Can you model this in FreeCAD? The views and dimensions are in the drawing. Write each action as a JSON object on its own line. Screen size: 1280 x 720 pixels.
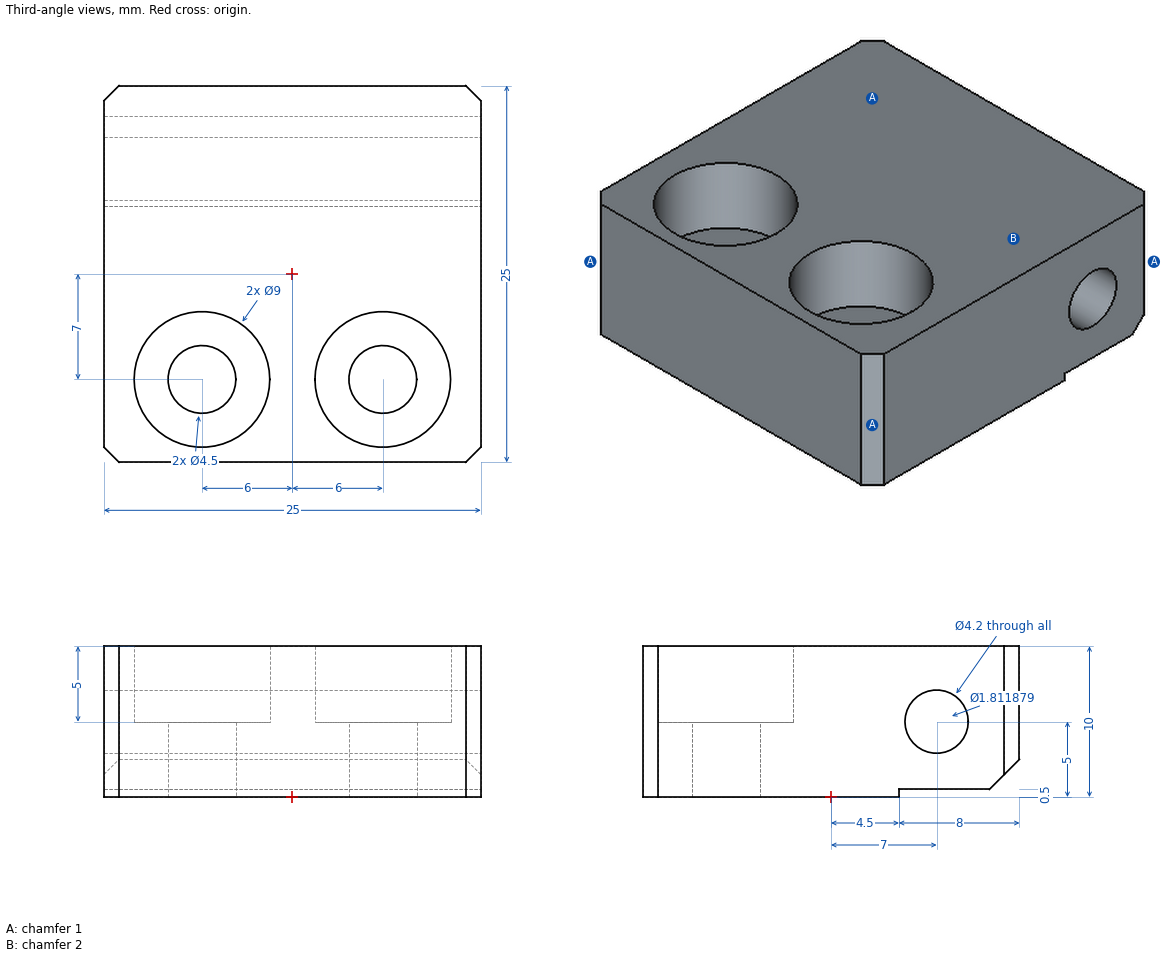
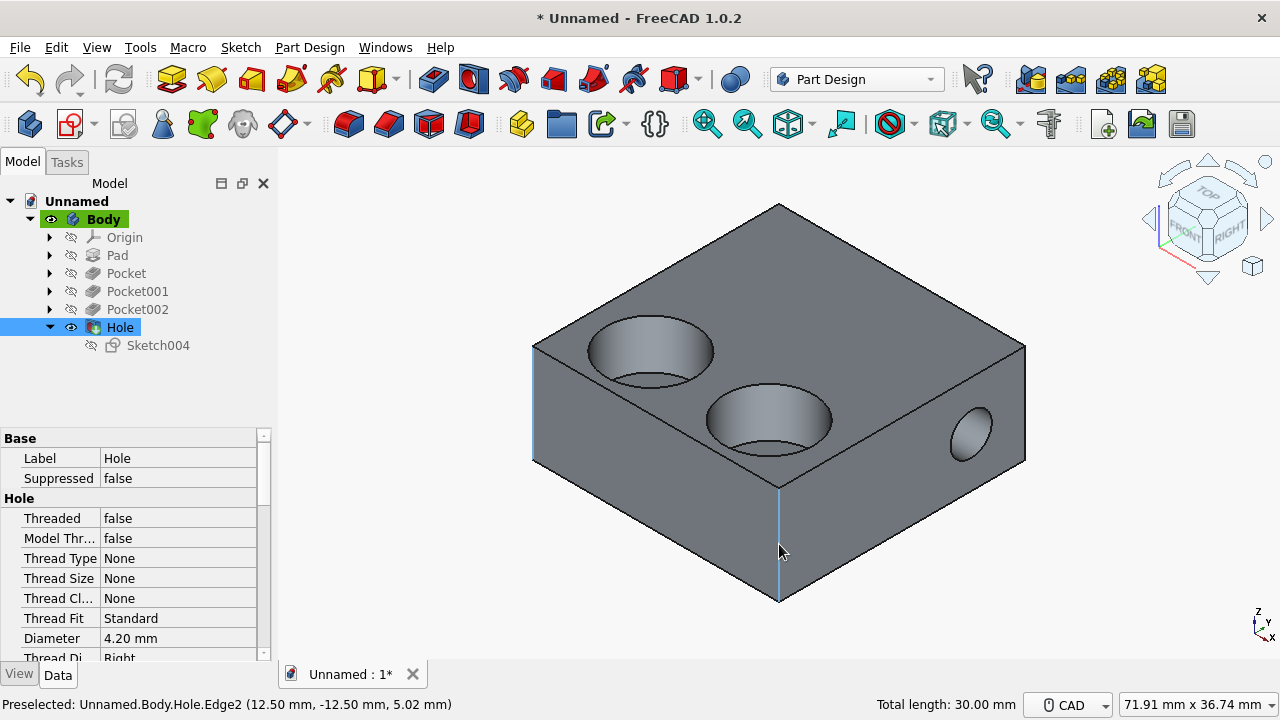
{"action": "key", "text": "2"}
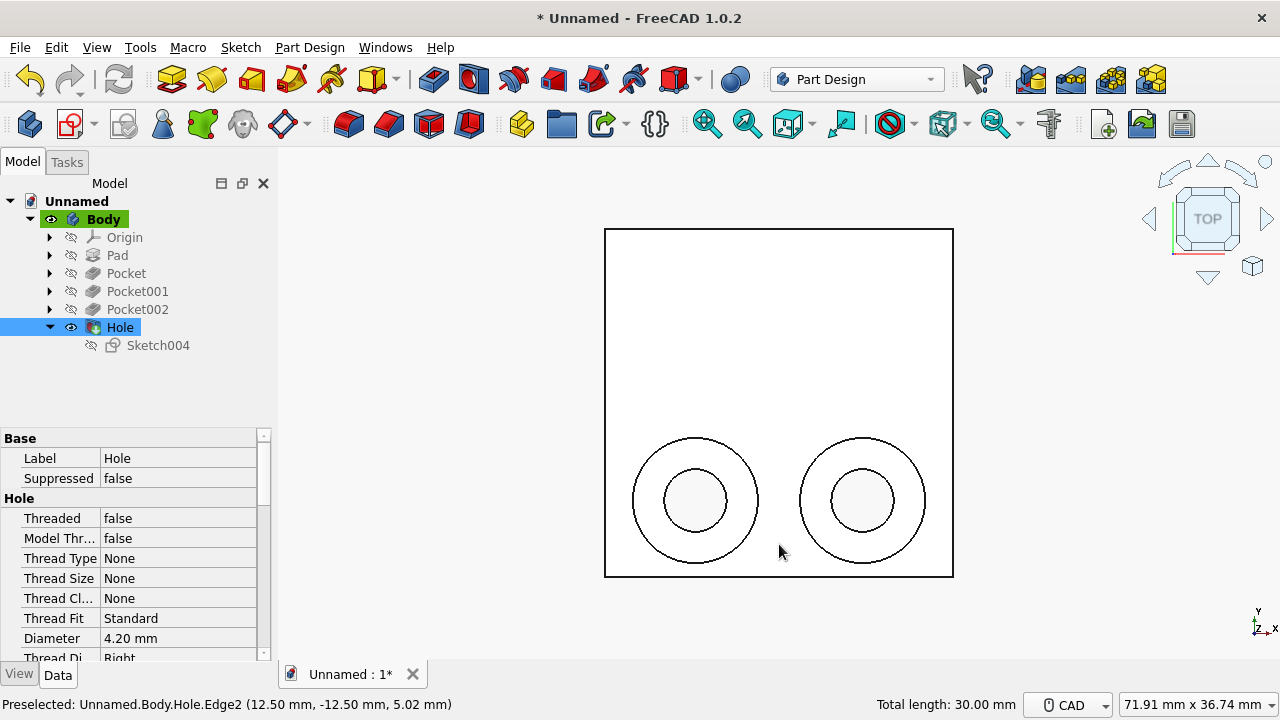
{"action": "key", "text": "1"}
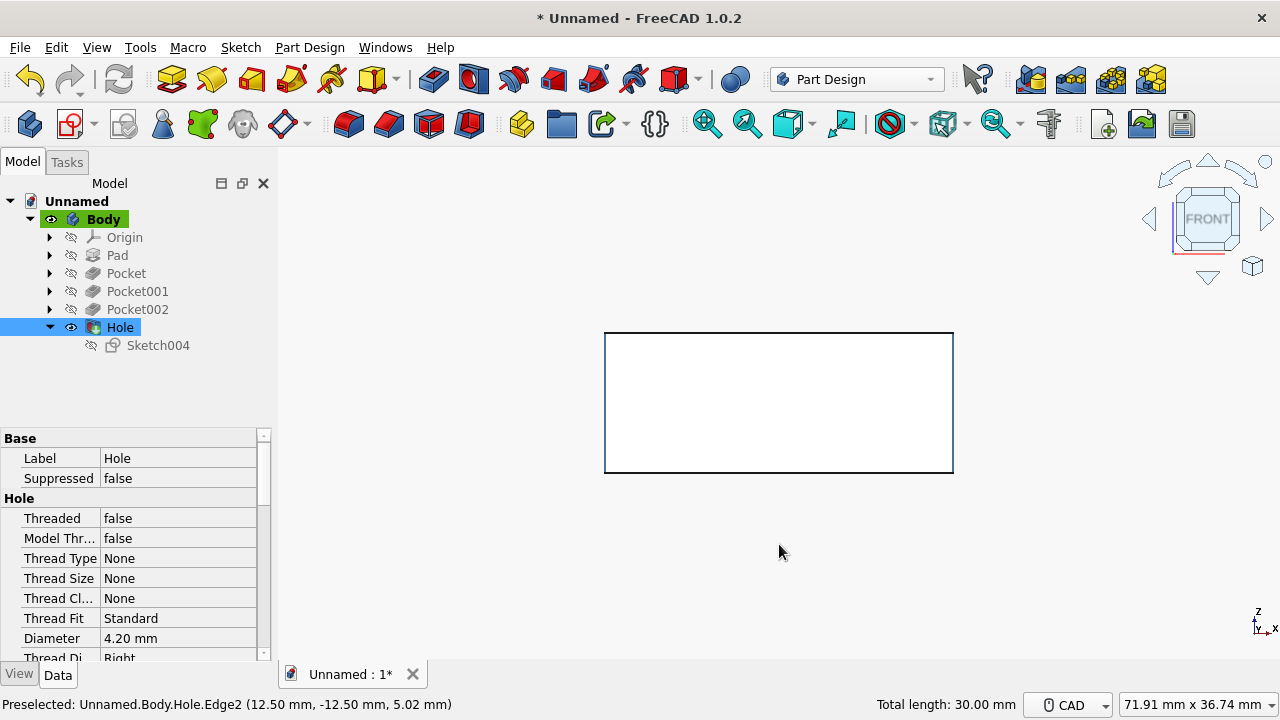
{"action": "key", "text": "v f"}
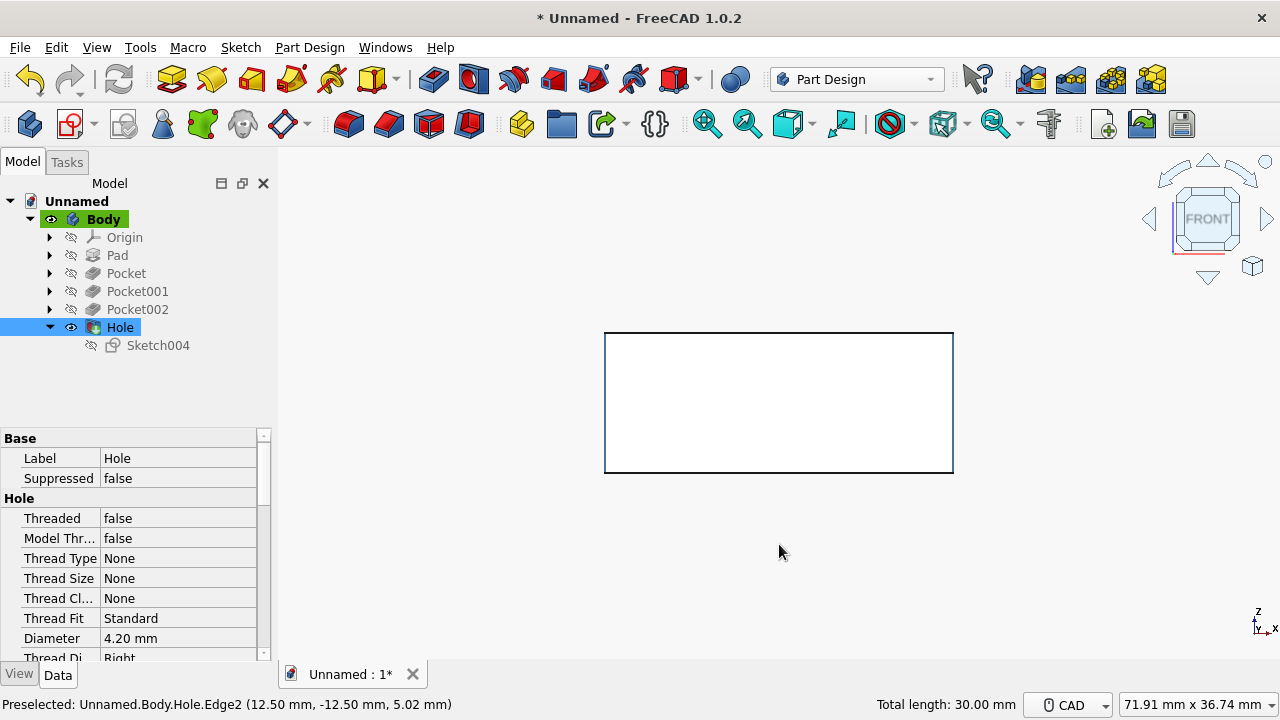
{"action": "key", "text": "3"}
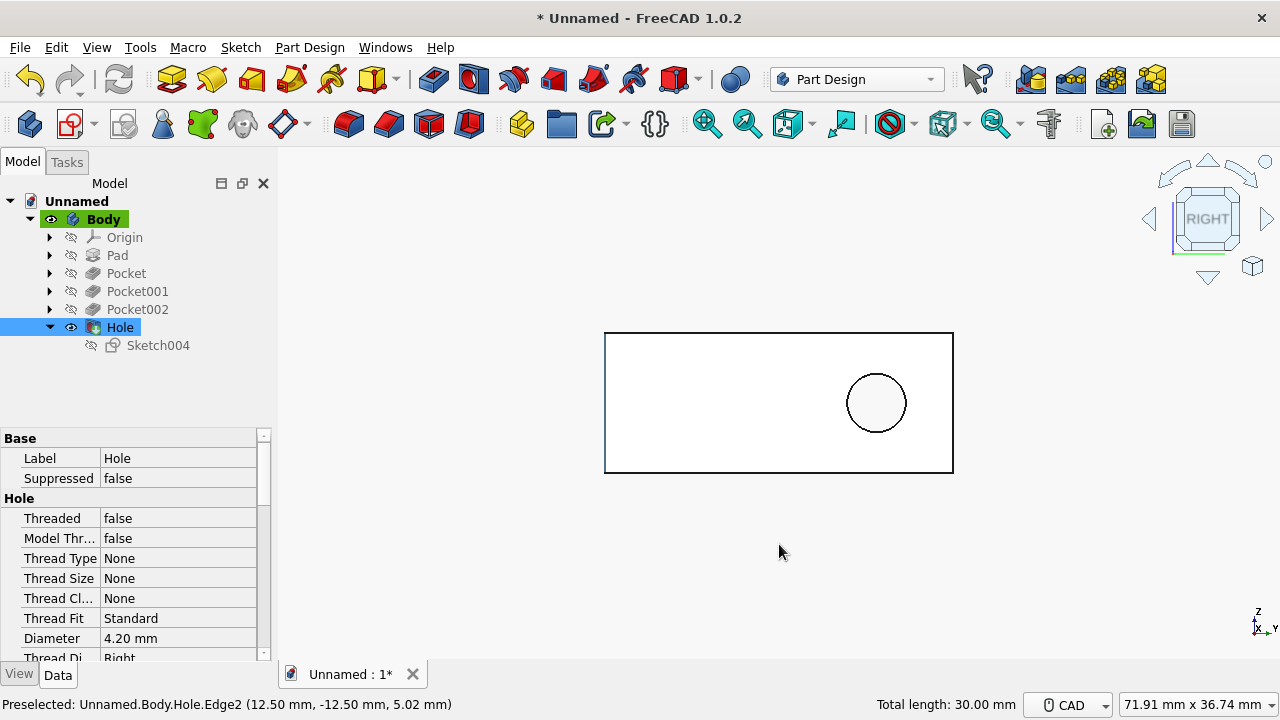
{"action": "key", "text": "v f"}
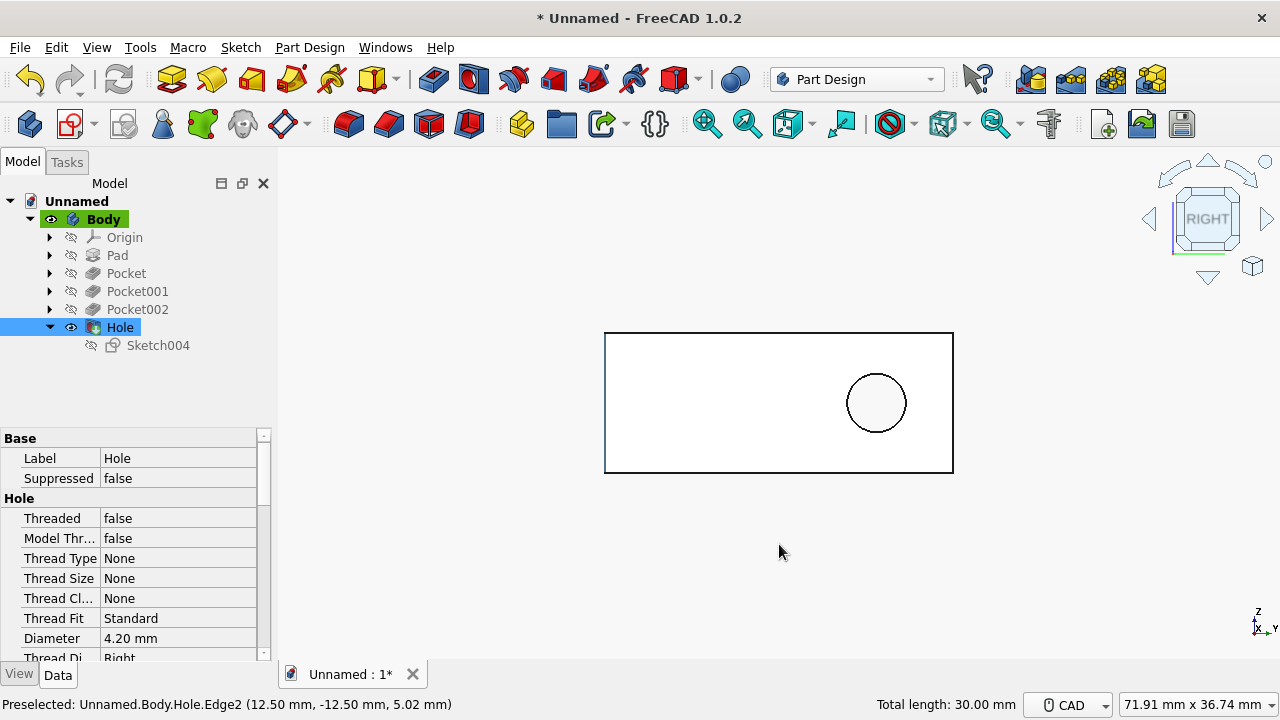
{"action": "left_click", "coordinate": [953, 402], "text": "ctrl"}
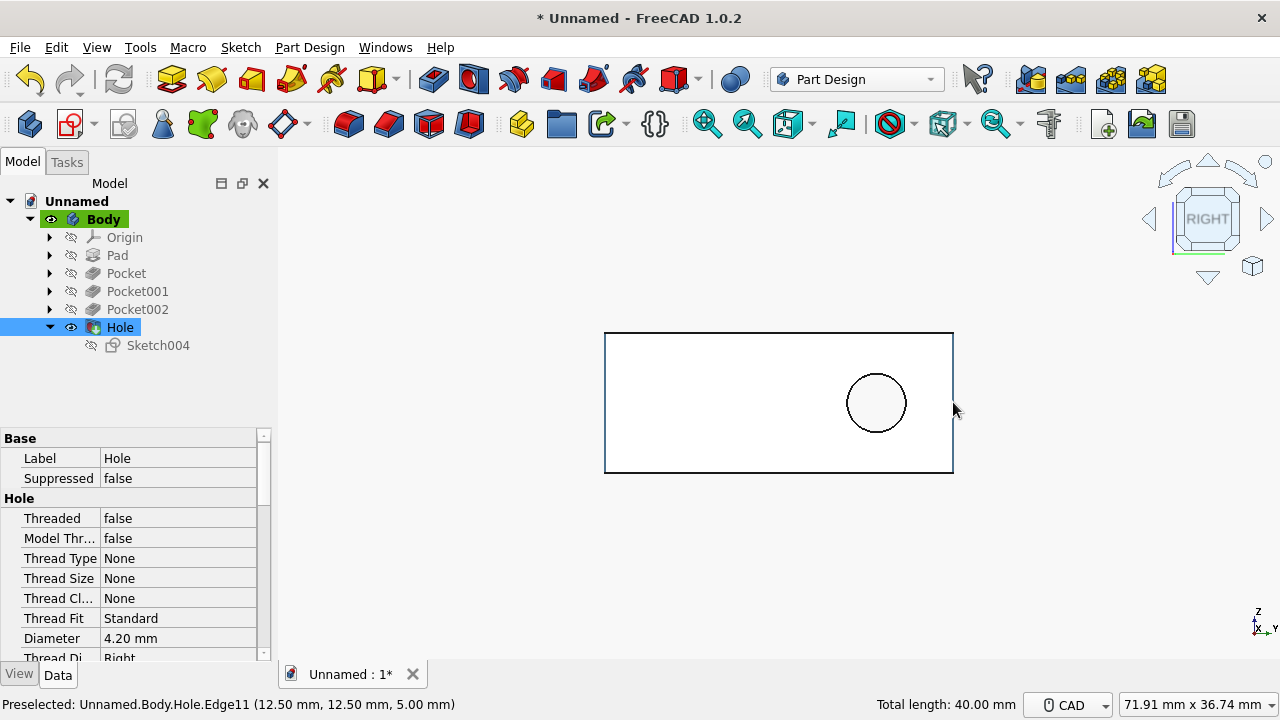
{"action": "left_click", "coordinate": [390, 124]}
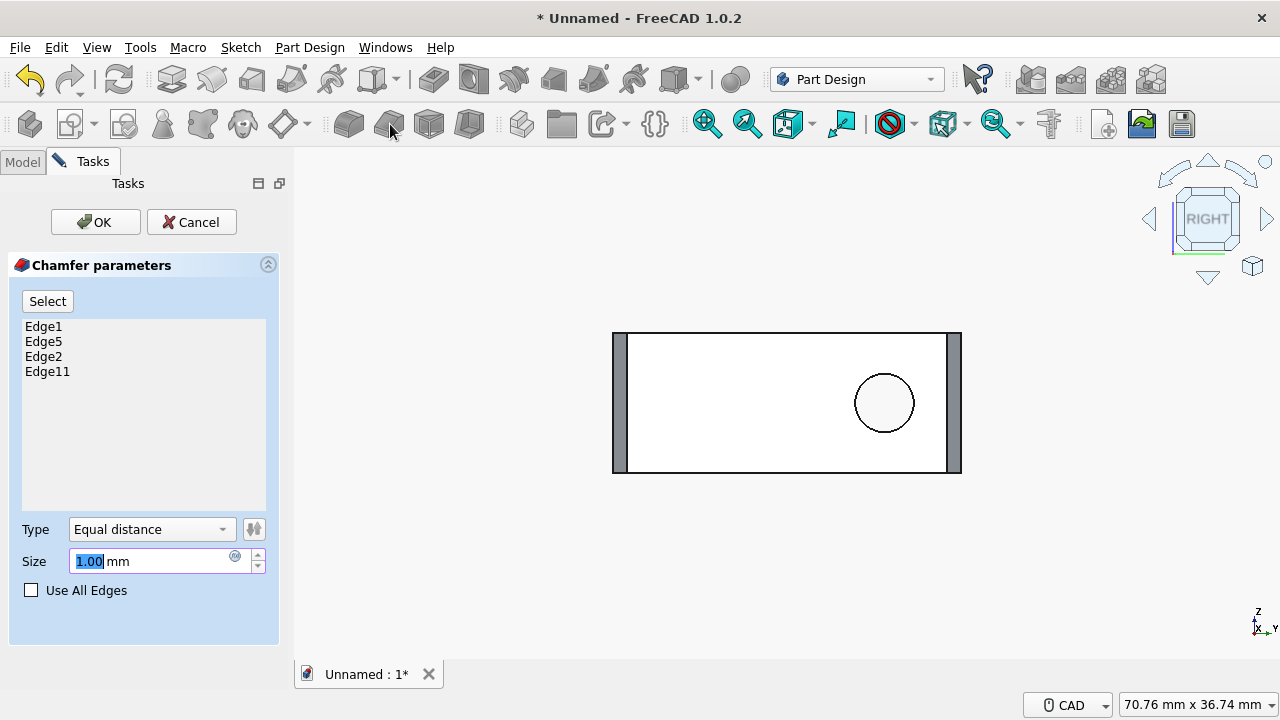
{"action": "type", "text": "1"}
{"action": "key", "text": "Tab"}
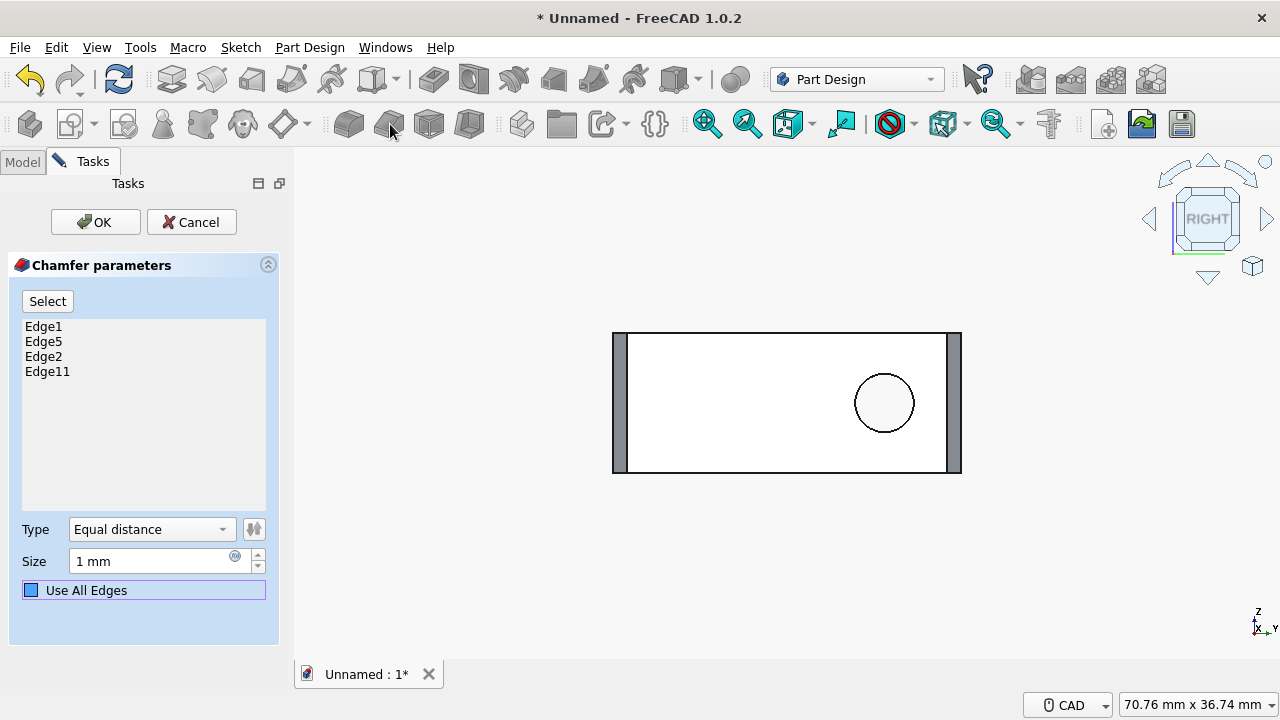
{"action": "left_click", "coordinate": [96, 222]}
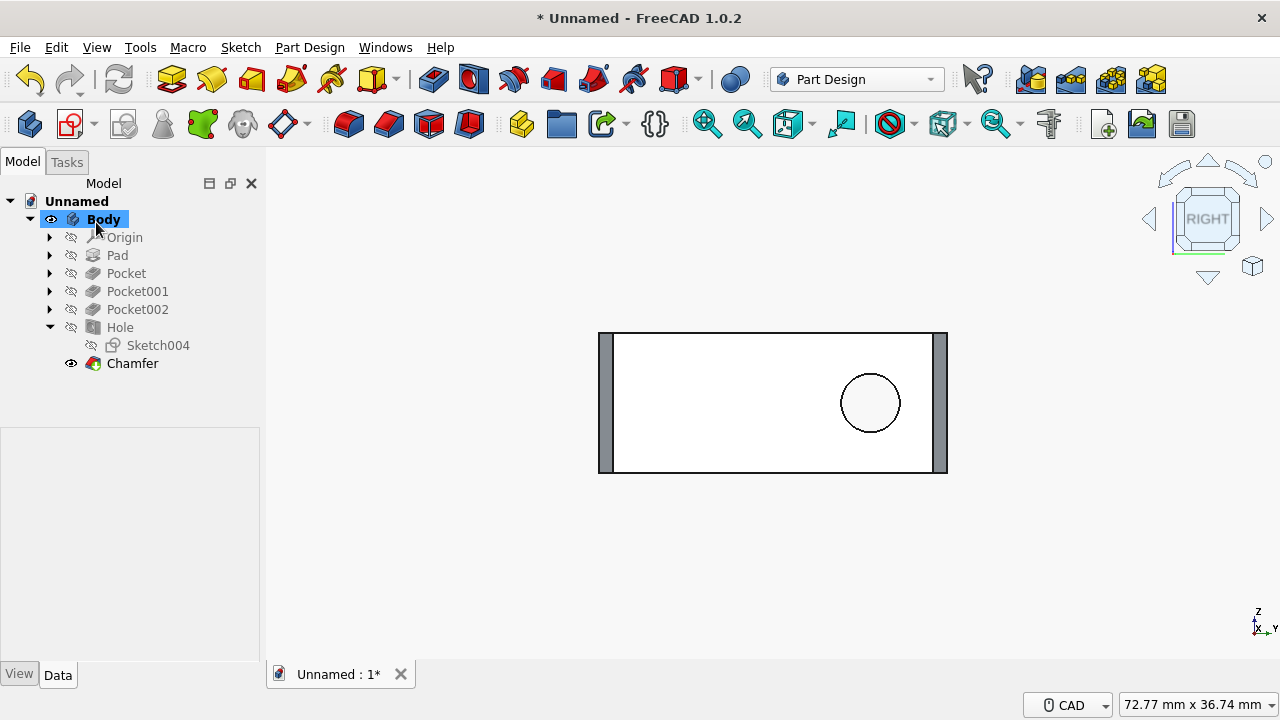
{"action": "left_click", "coordinate": [708, 124]}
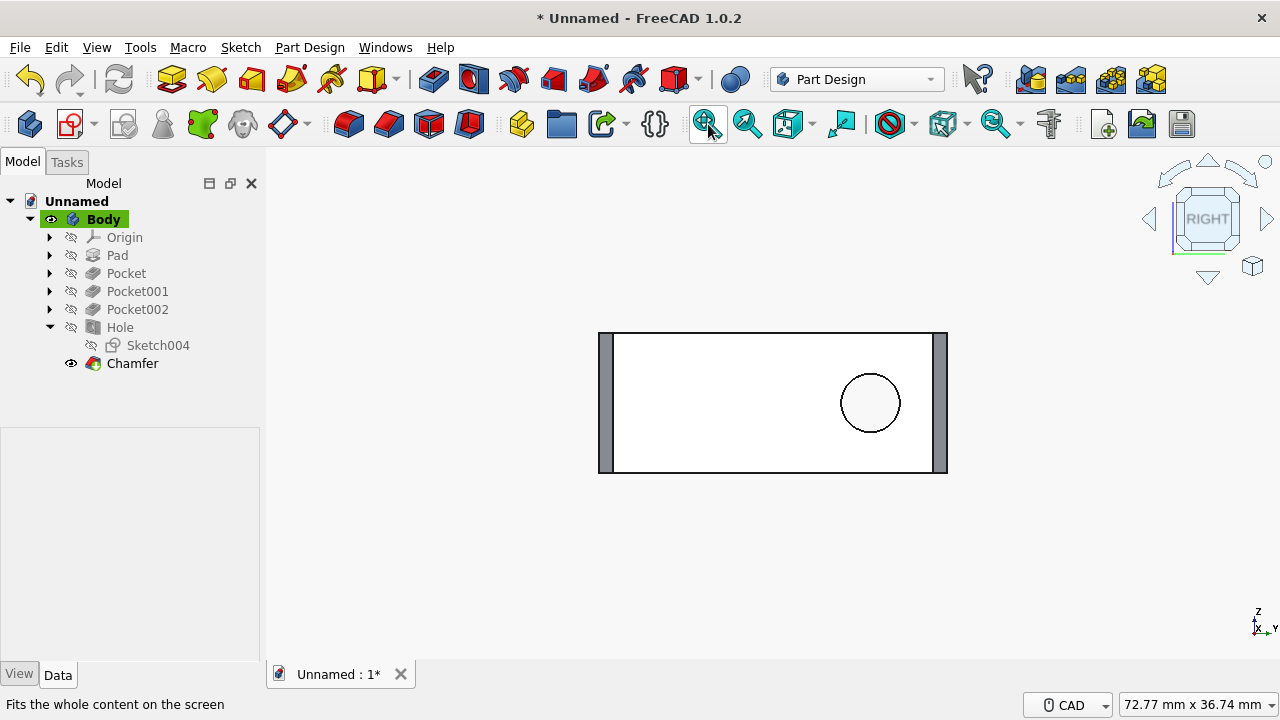
{"action": "key", "text": "6"}